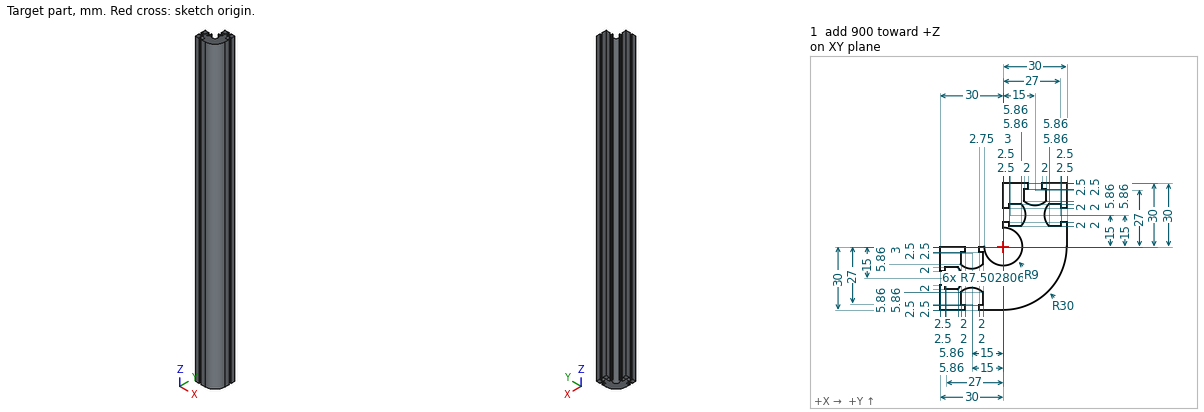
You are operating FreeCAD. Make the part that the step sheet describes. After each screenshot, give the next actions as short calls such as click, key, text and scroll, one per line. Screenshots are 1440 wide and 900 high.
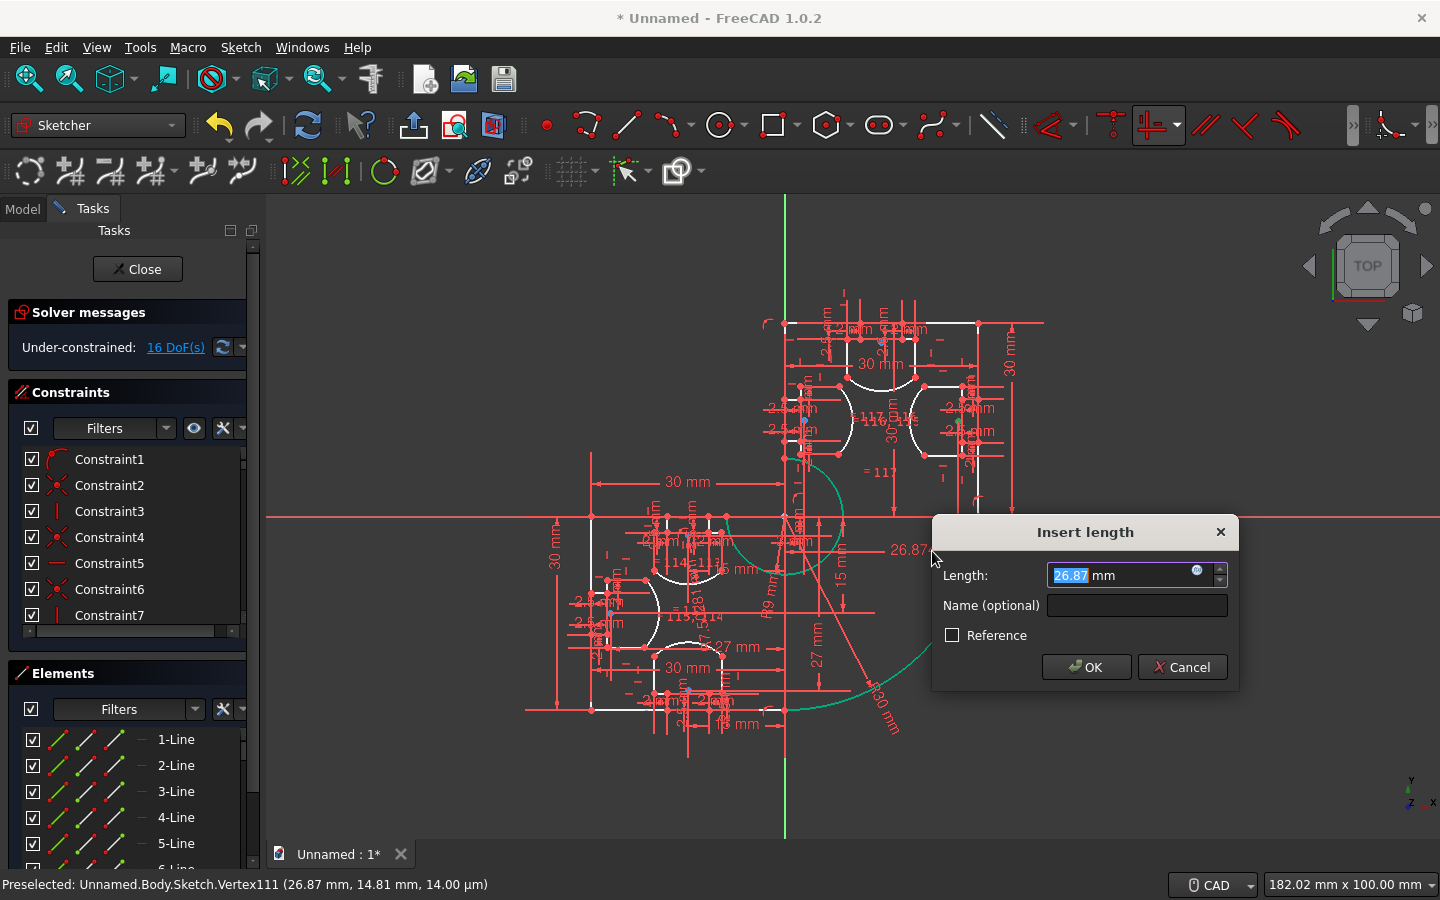
text(27)
key(Return)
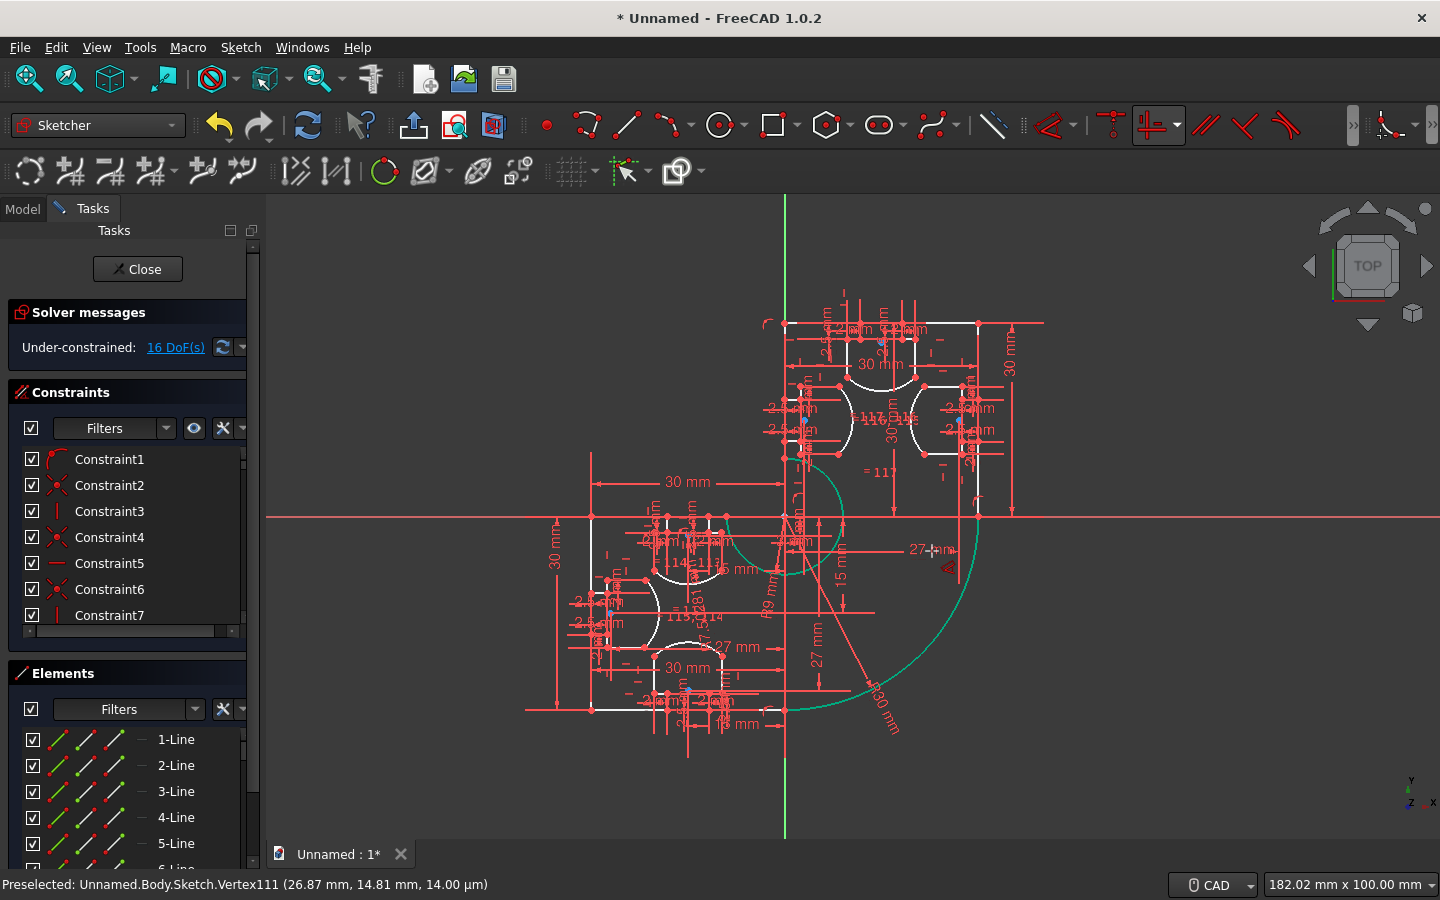
click(959, 421)
click(993, 469)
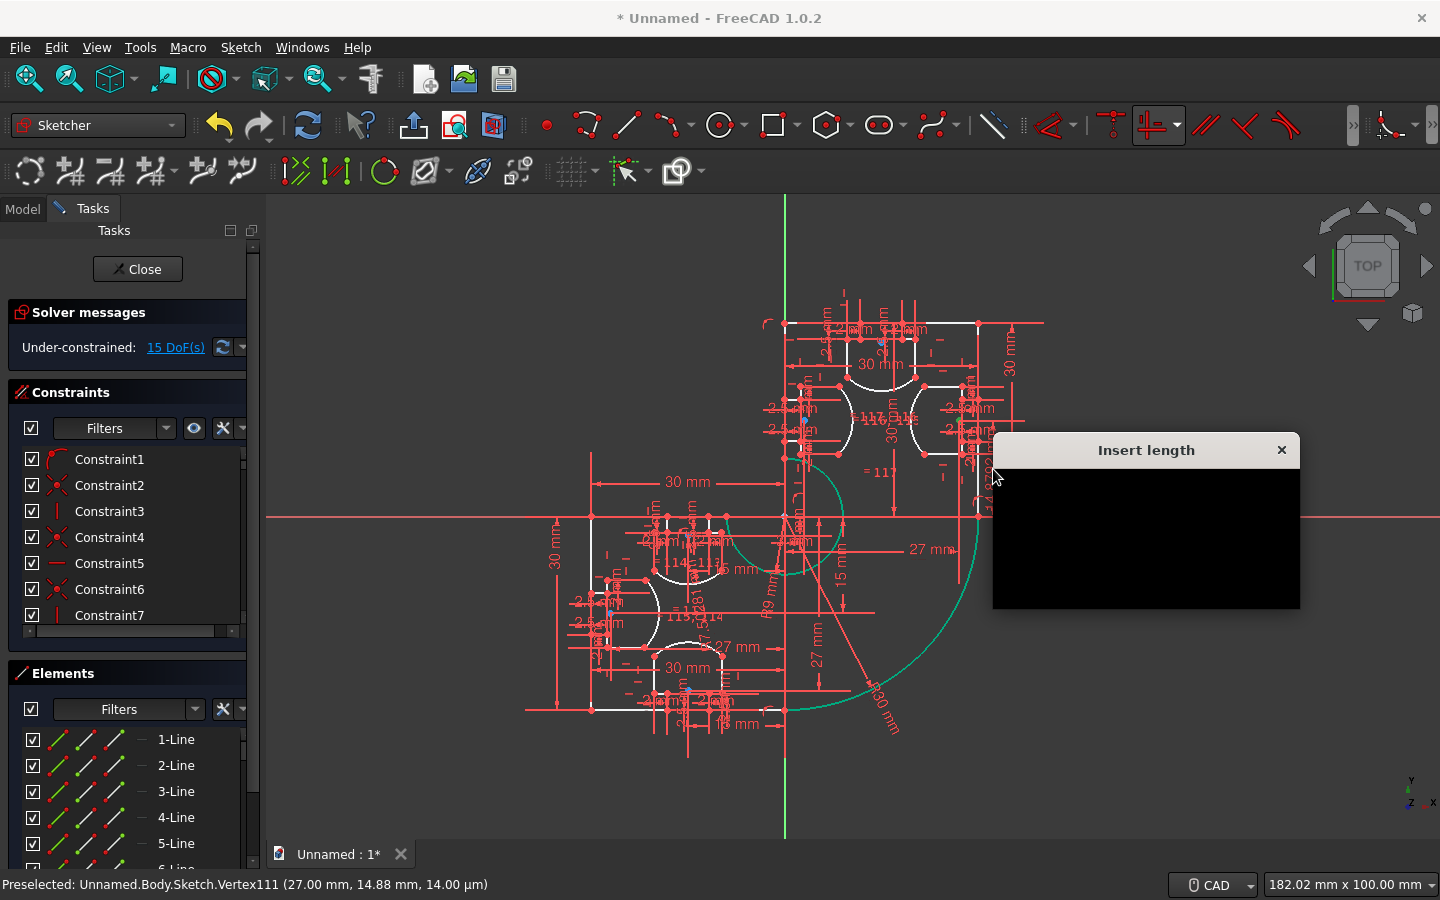
text(15)
key(Return)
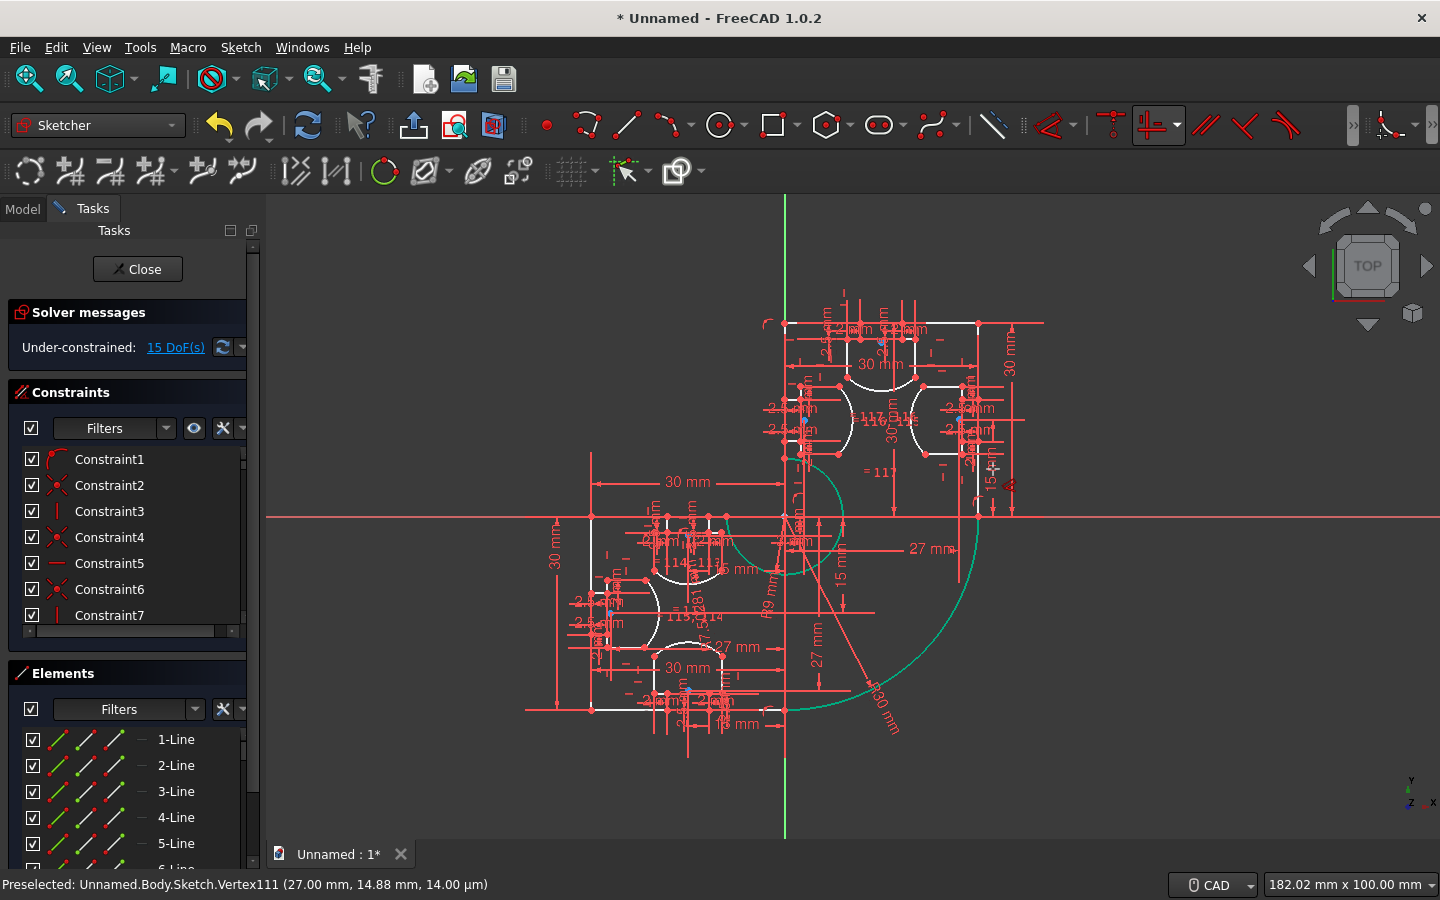
click(881, 343)
click(833, 309)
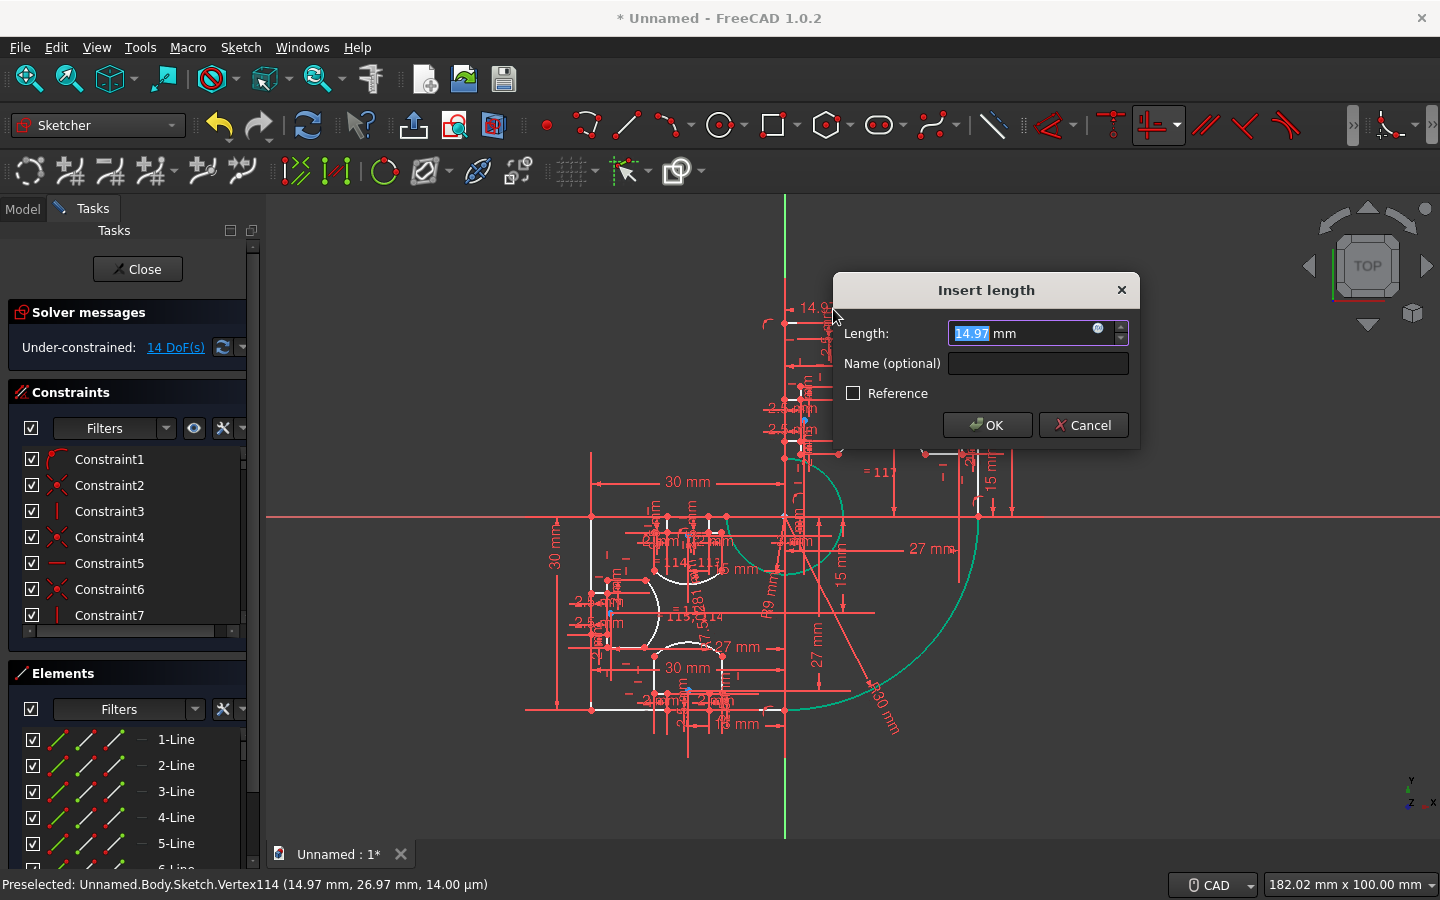
text(15)
key(Return)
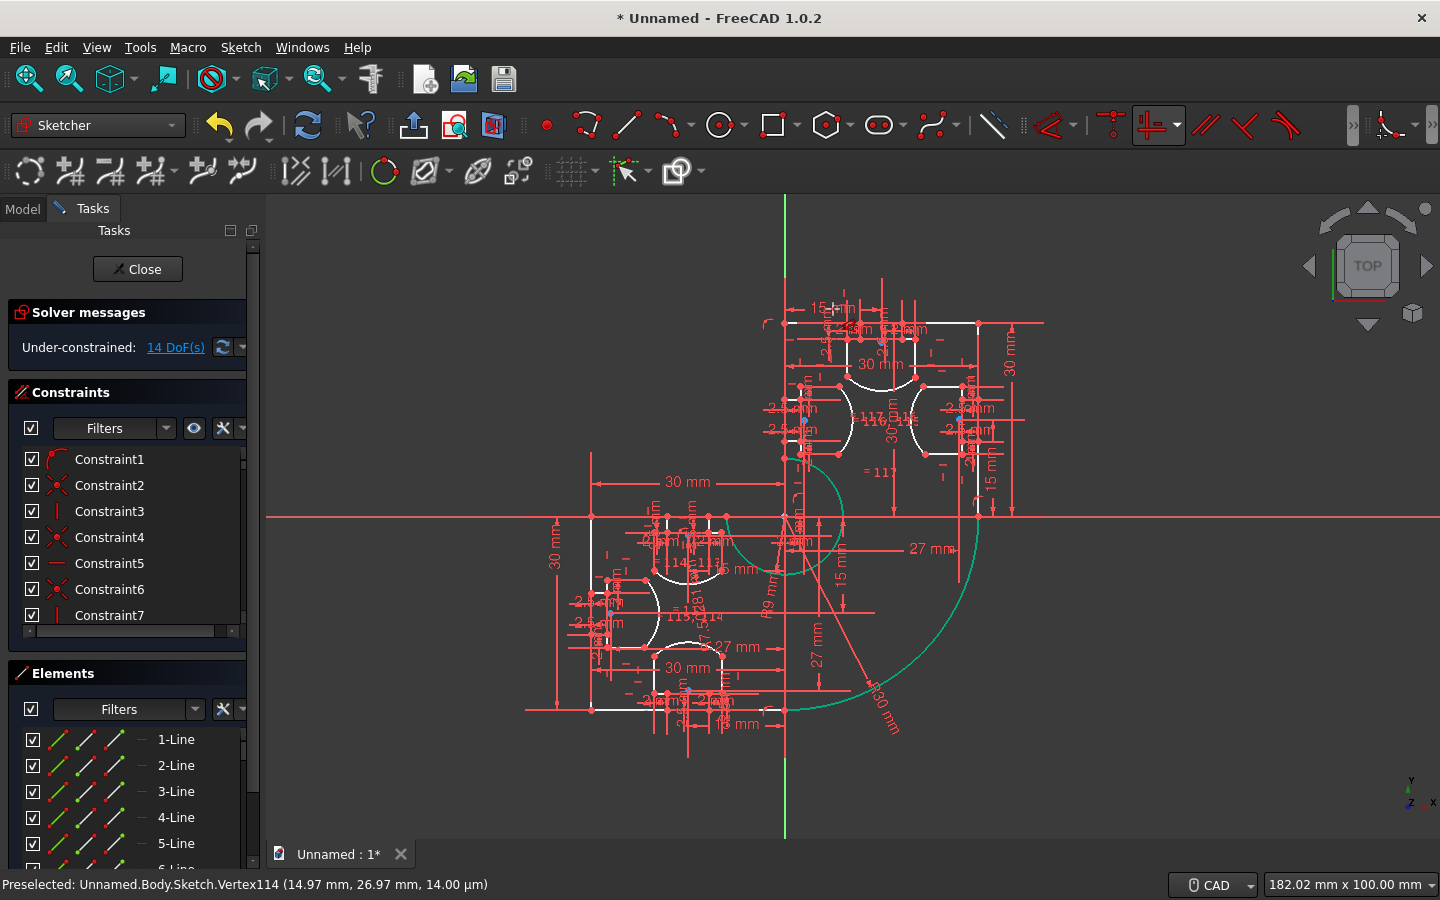
click(882, 342)
click(916, 470)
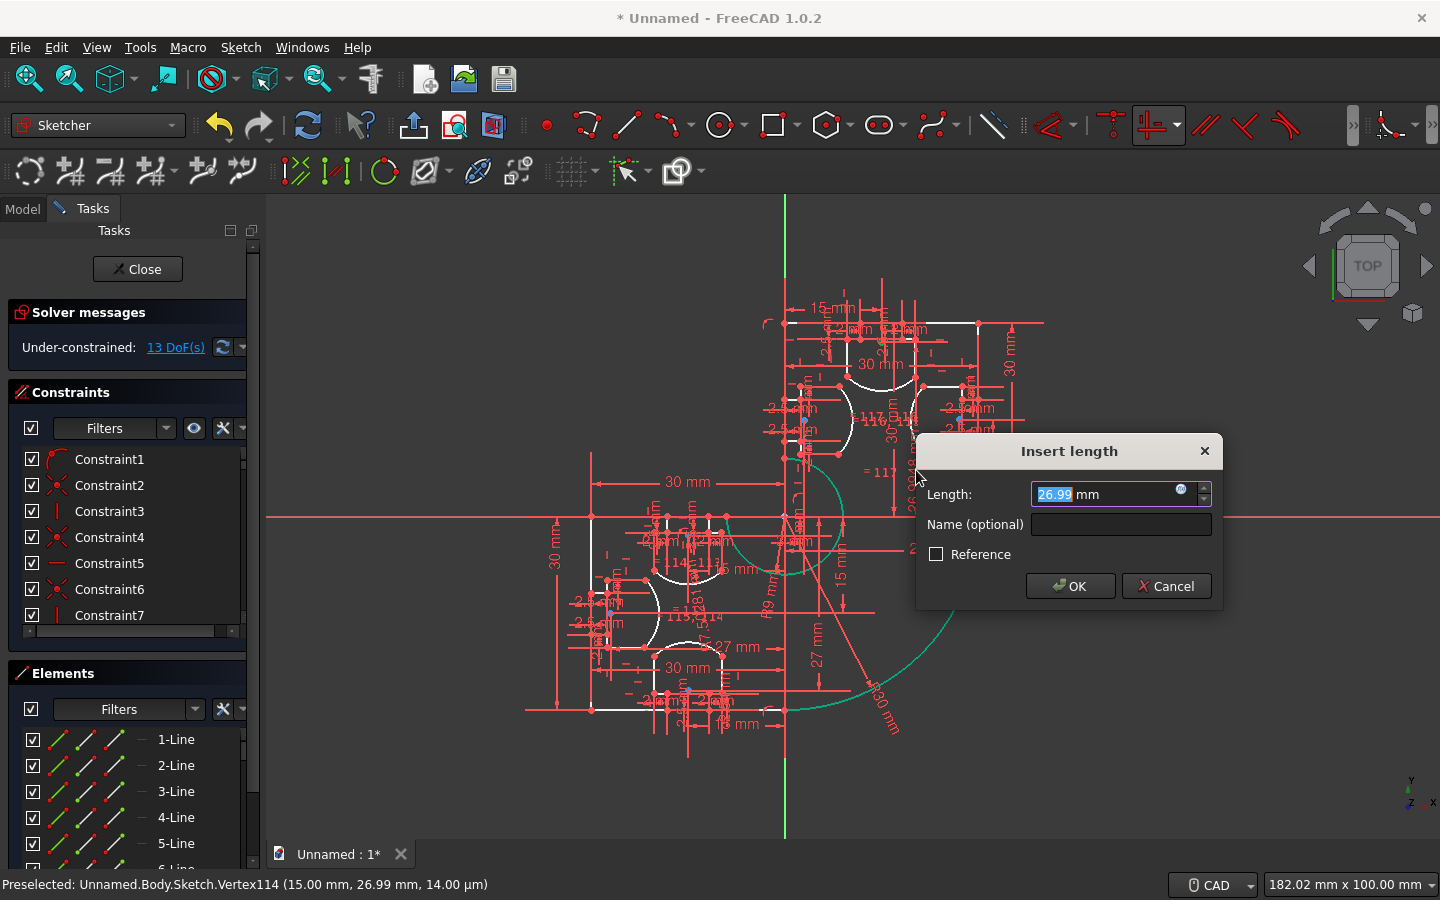
text(27)
key(Return)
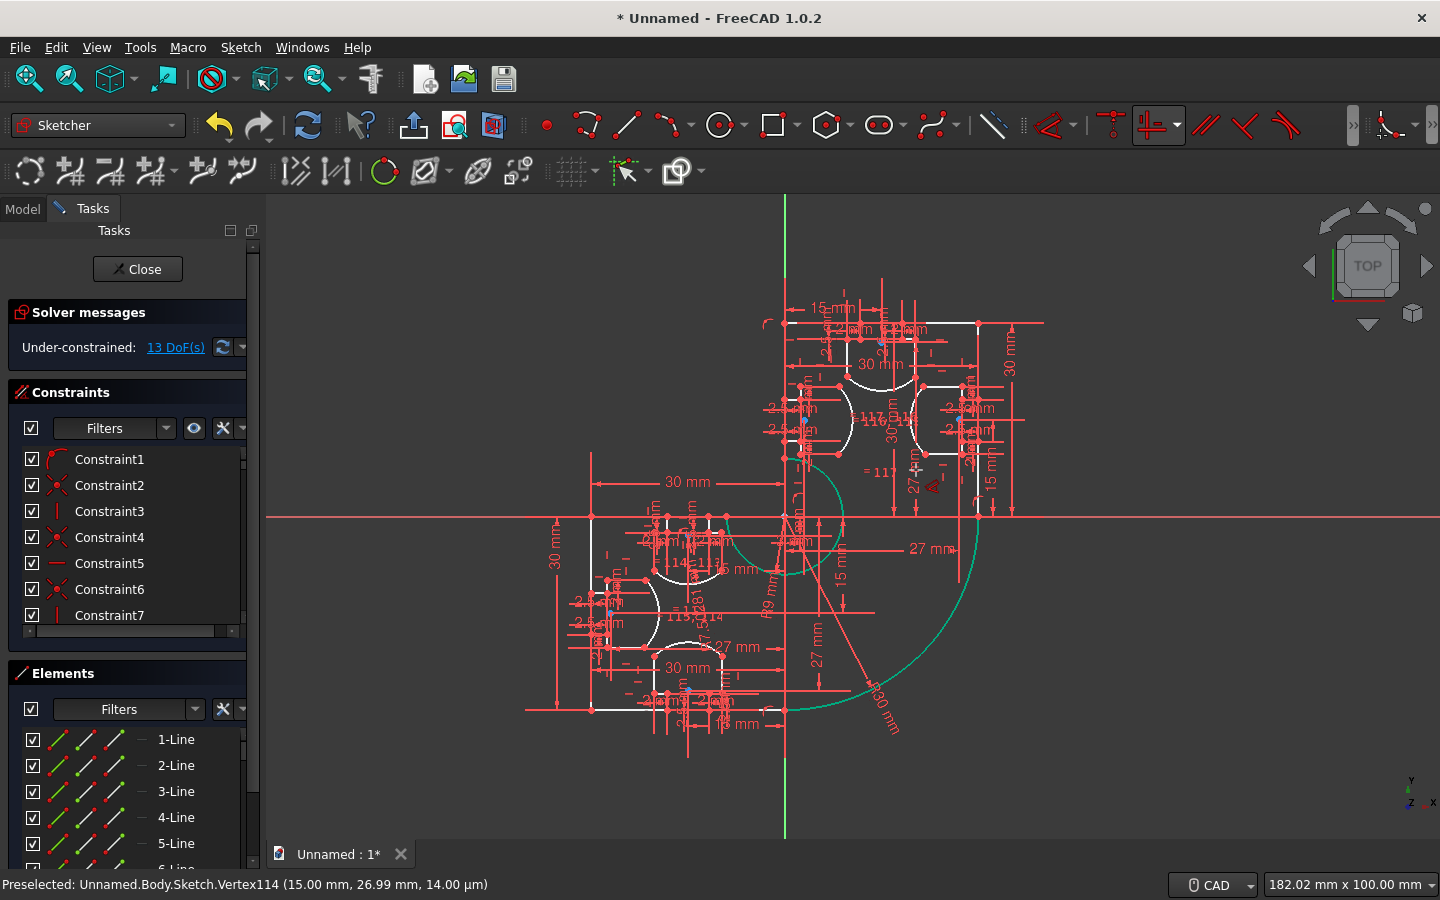
click(804, 420)
click(838, 468)